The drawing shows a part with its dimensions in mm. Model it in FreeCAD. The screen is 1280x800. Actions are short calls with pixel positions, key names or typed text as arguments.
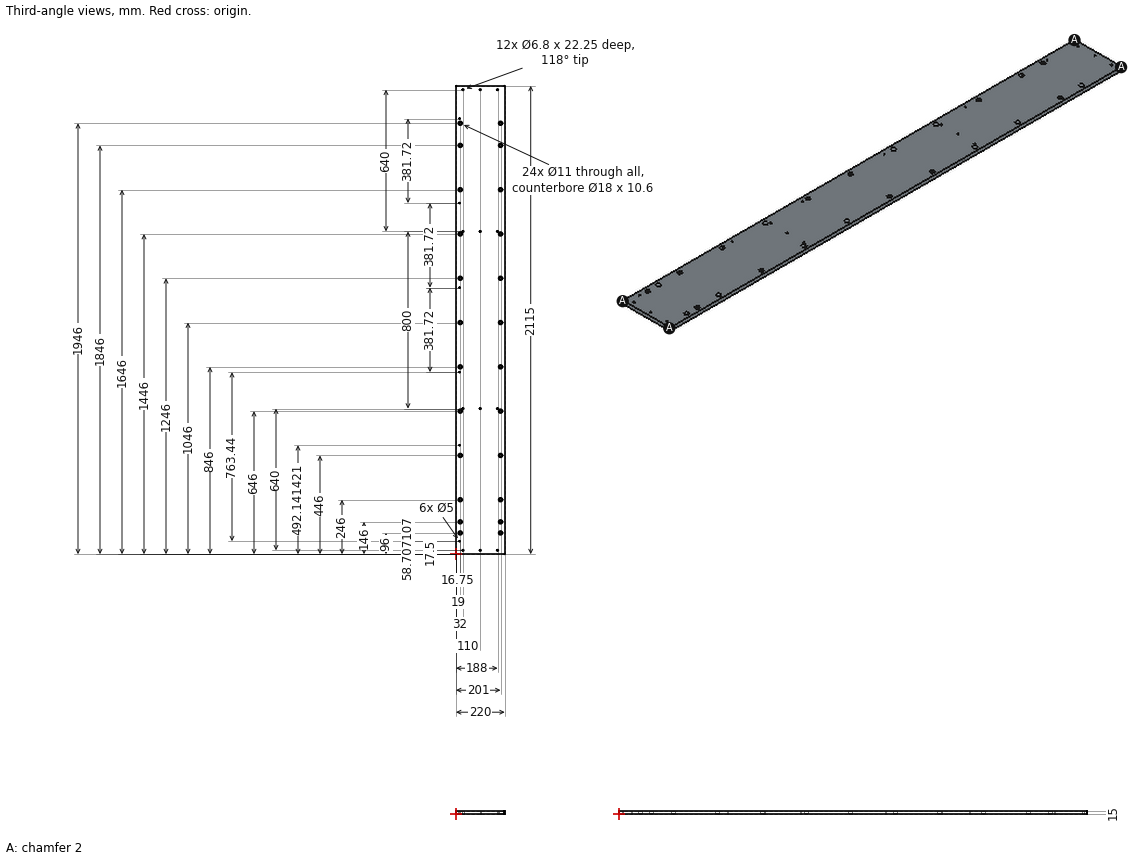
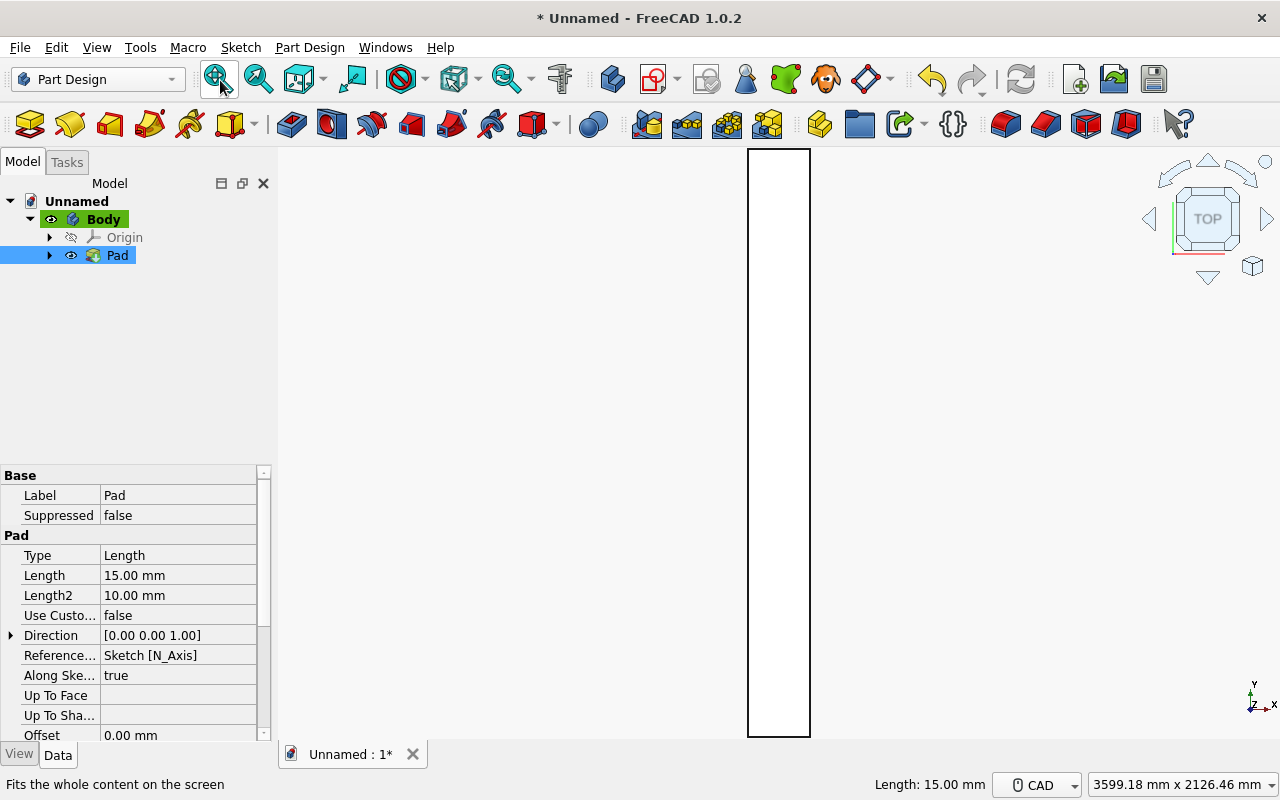
key(1)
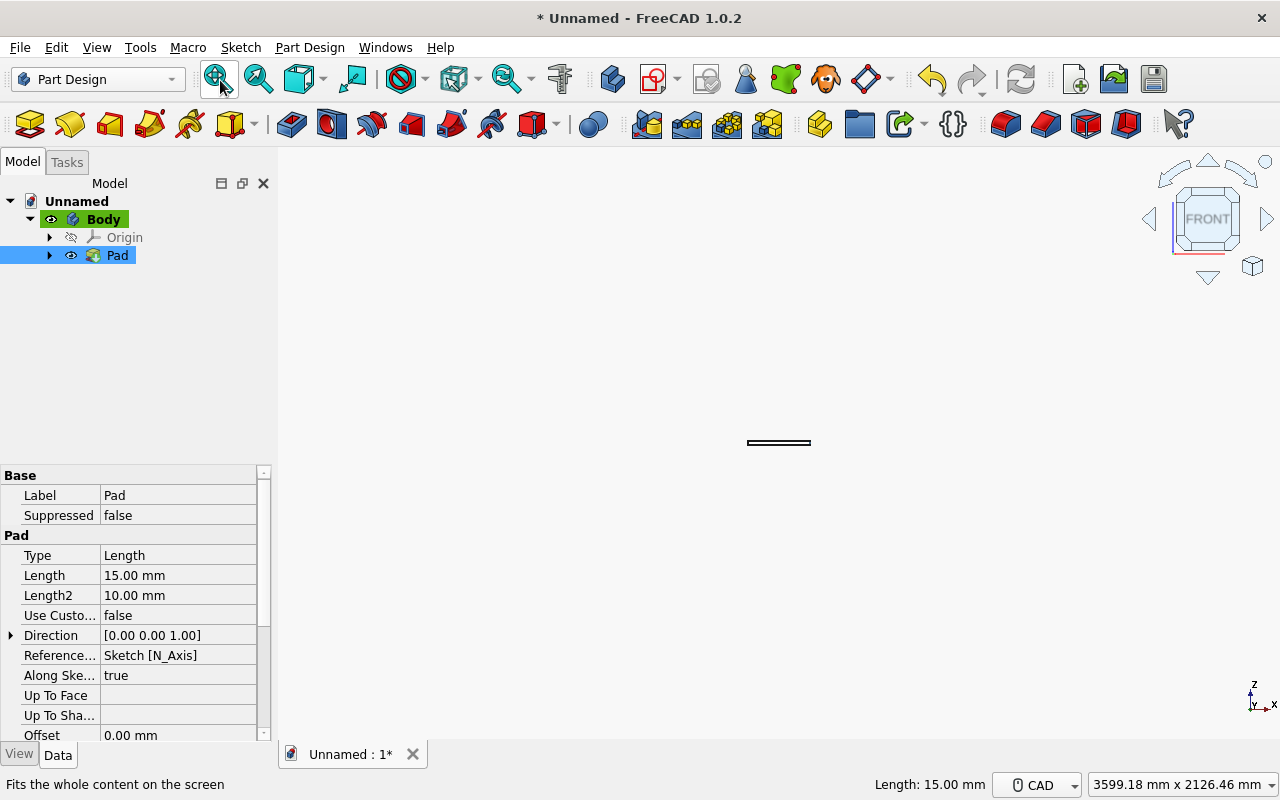
click(220, 80)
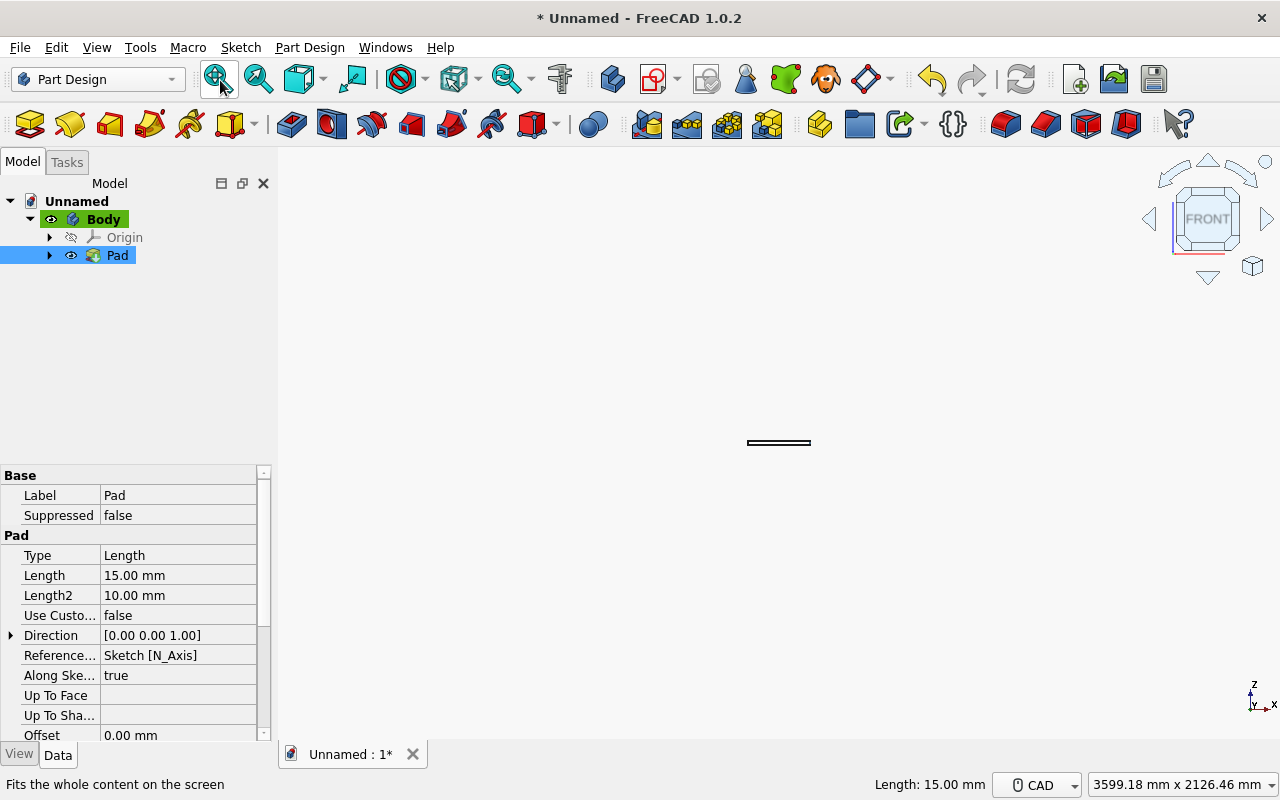
scroll(748, 442, up, 12)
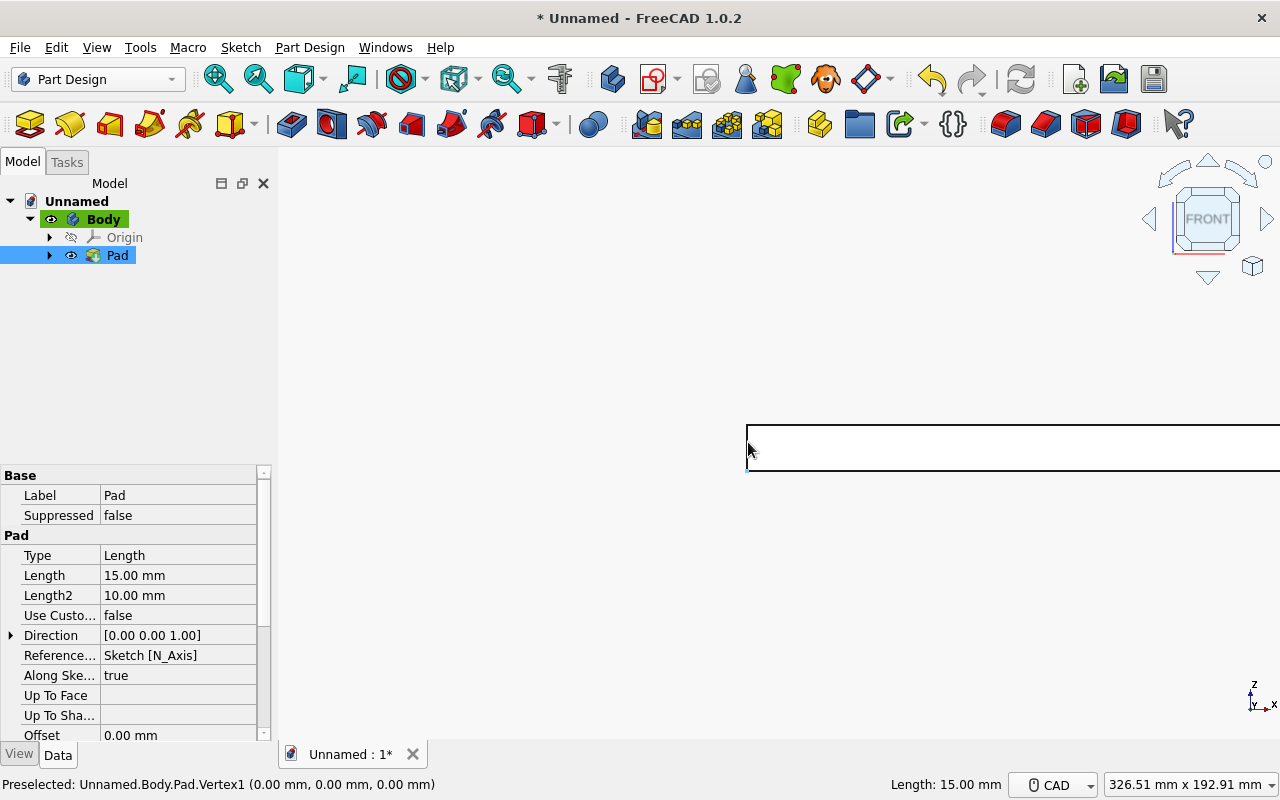
click(747, 447, ctrl)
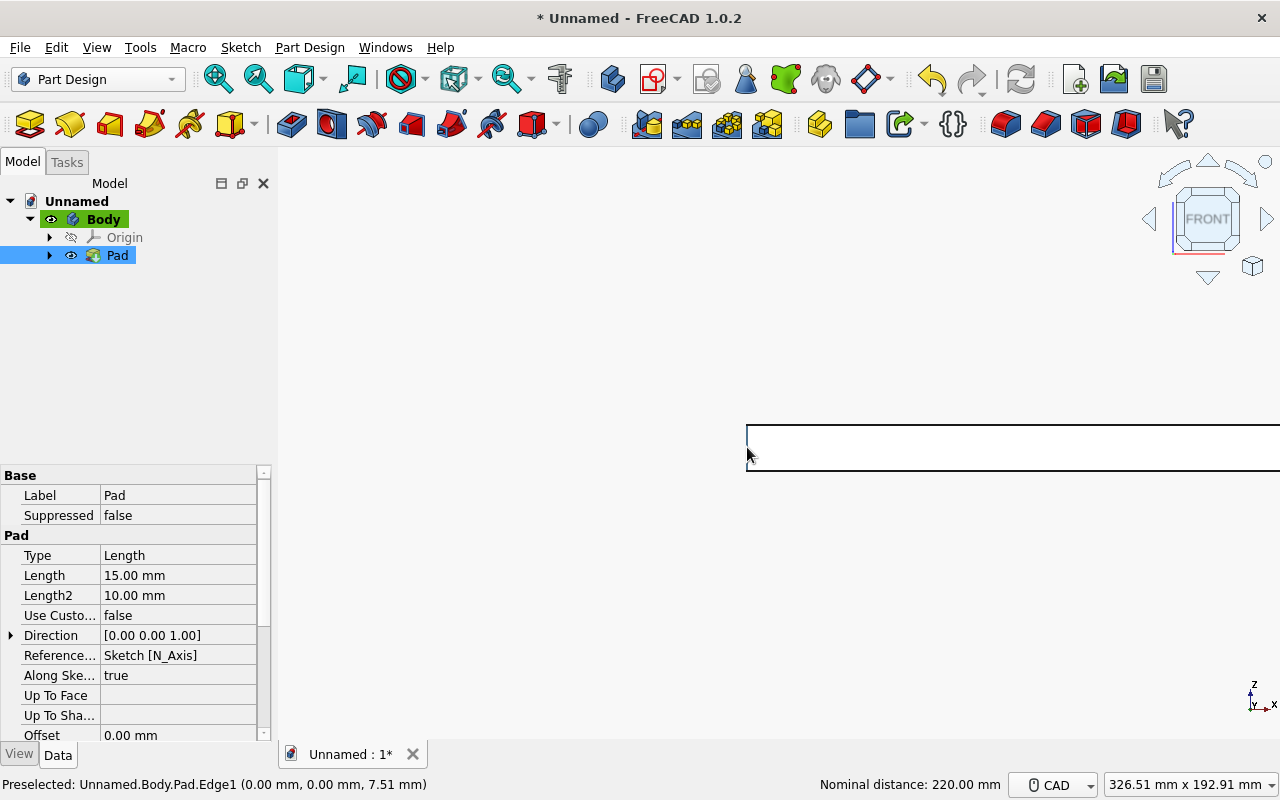
click(220, 80)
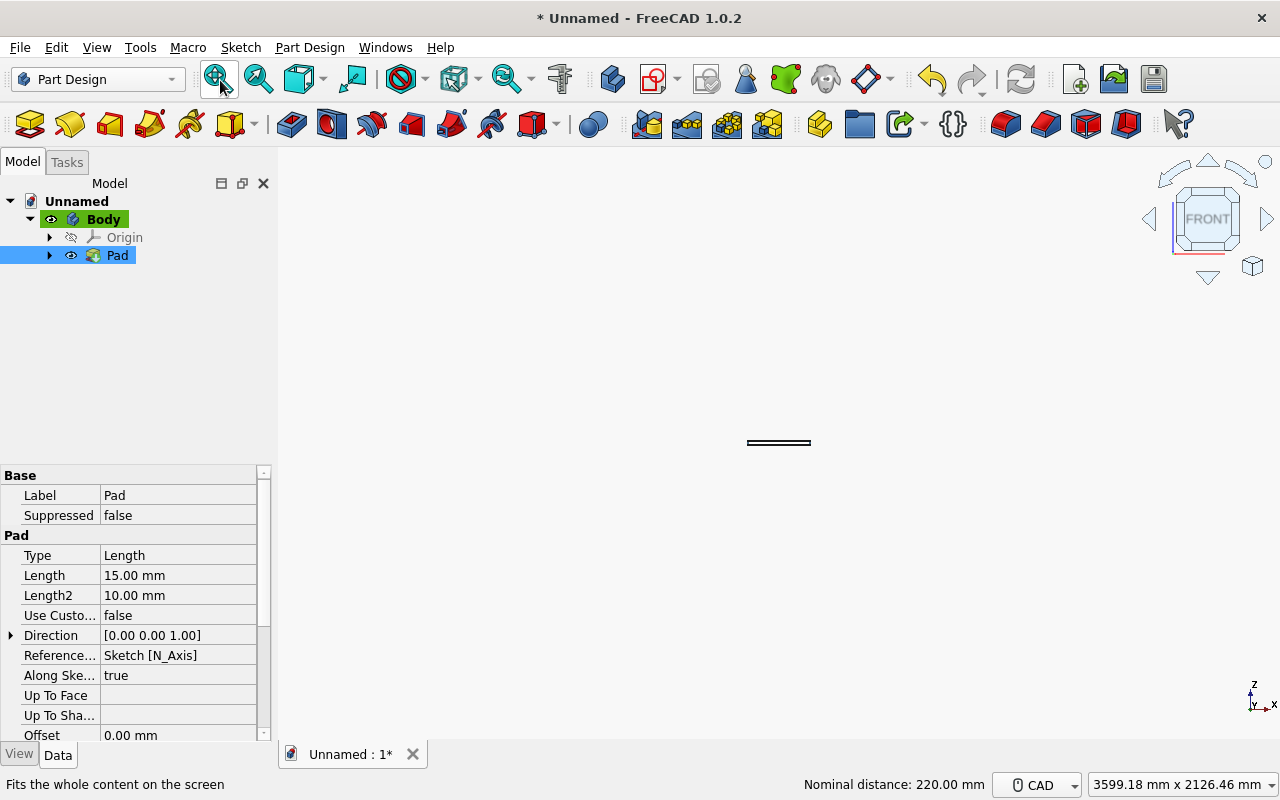
key(3)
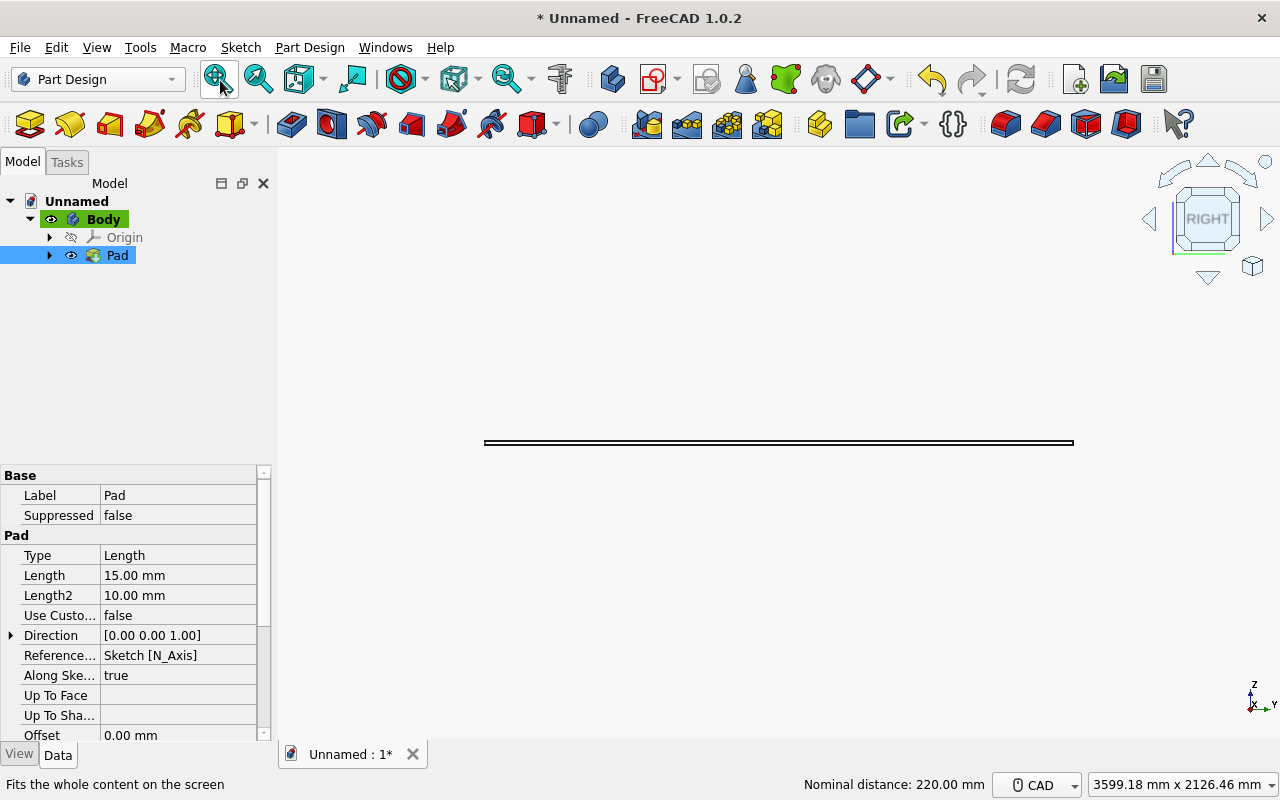
scroll(1073, 442, up, 12)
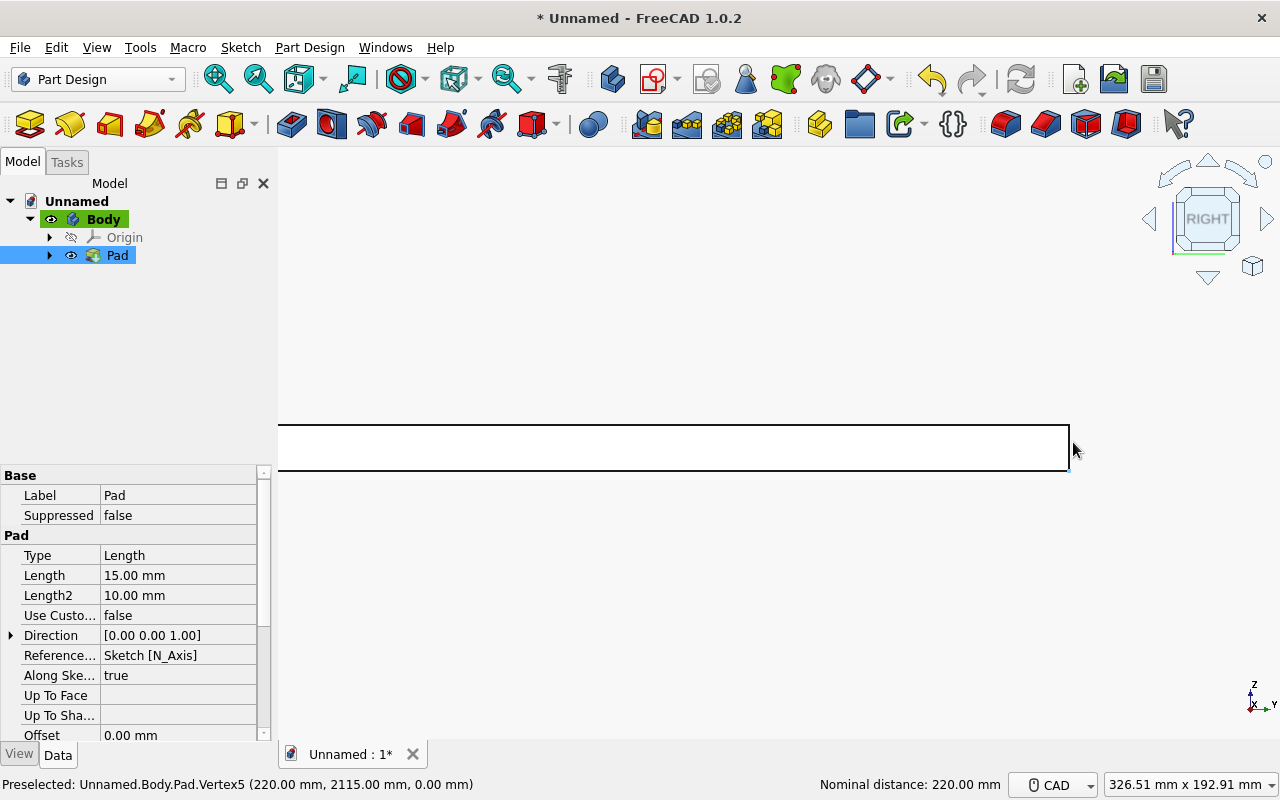
click(1069, 447, ctrl)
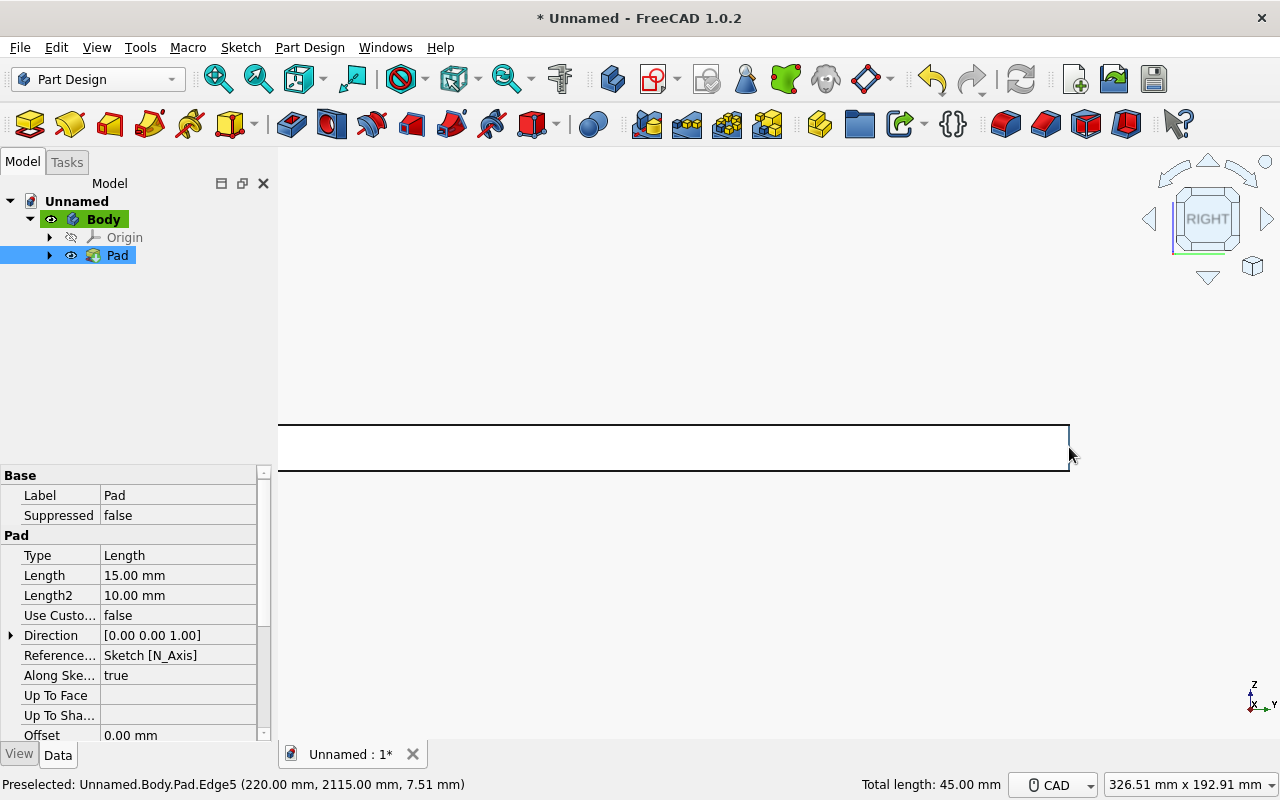
click(220, 80)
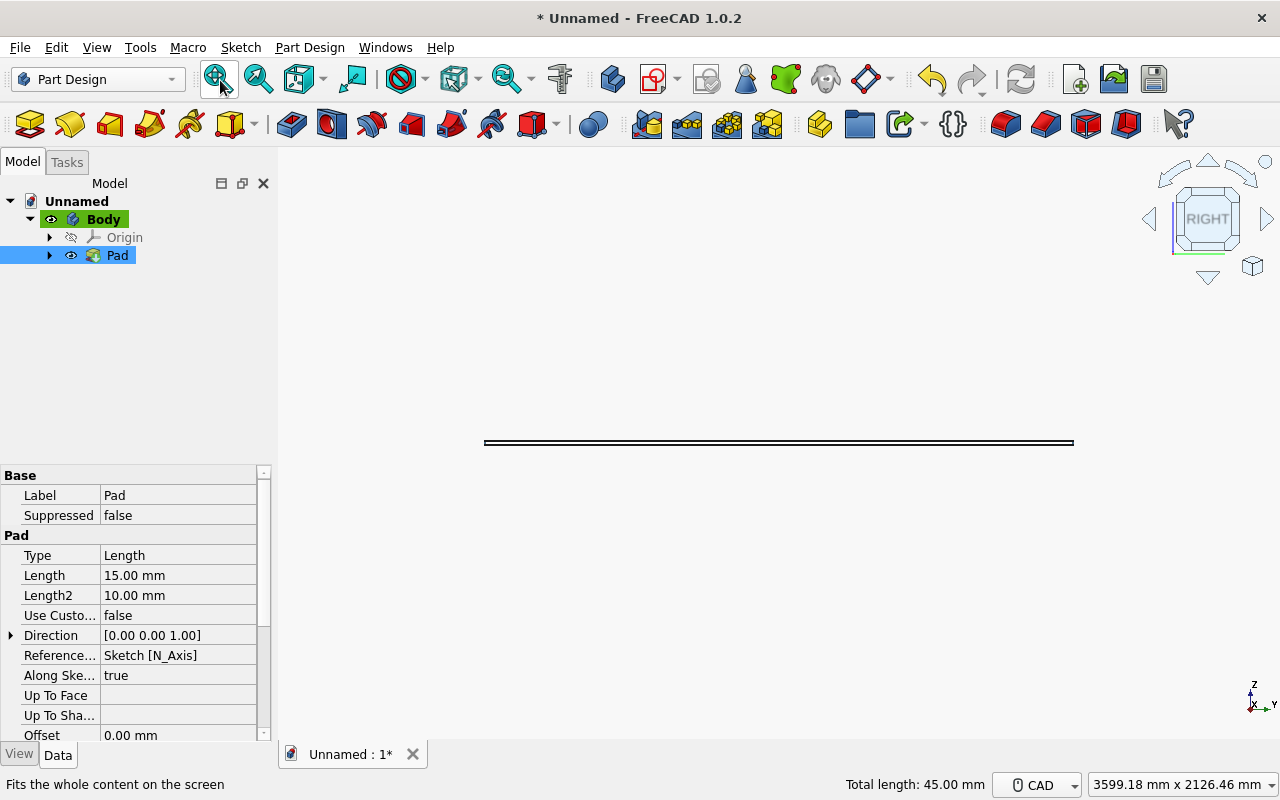
key(5)